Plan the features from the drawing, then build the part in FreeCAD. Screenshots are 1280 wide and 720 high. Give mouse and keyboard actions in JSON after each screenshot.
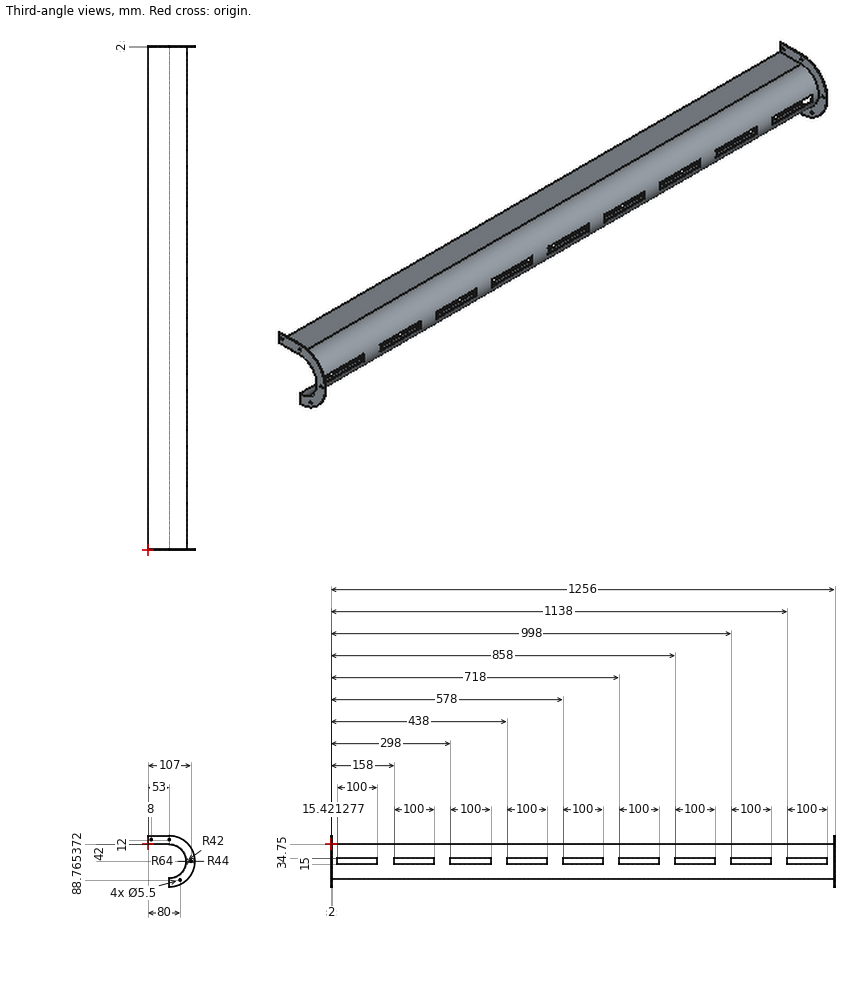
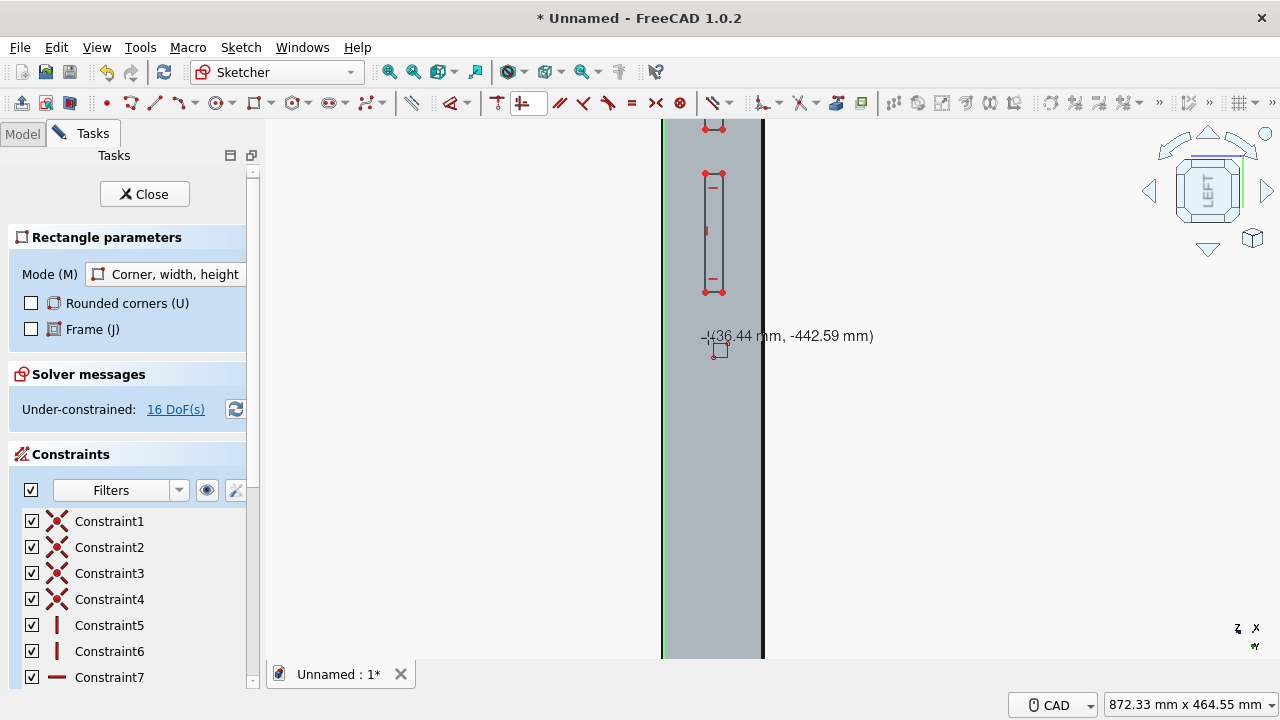
{"action": "left_click", "coordinate": [705, 335]}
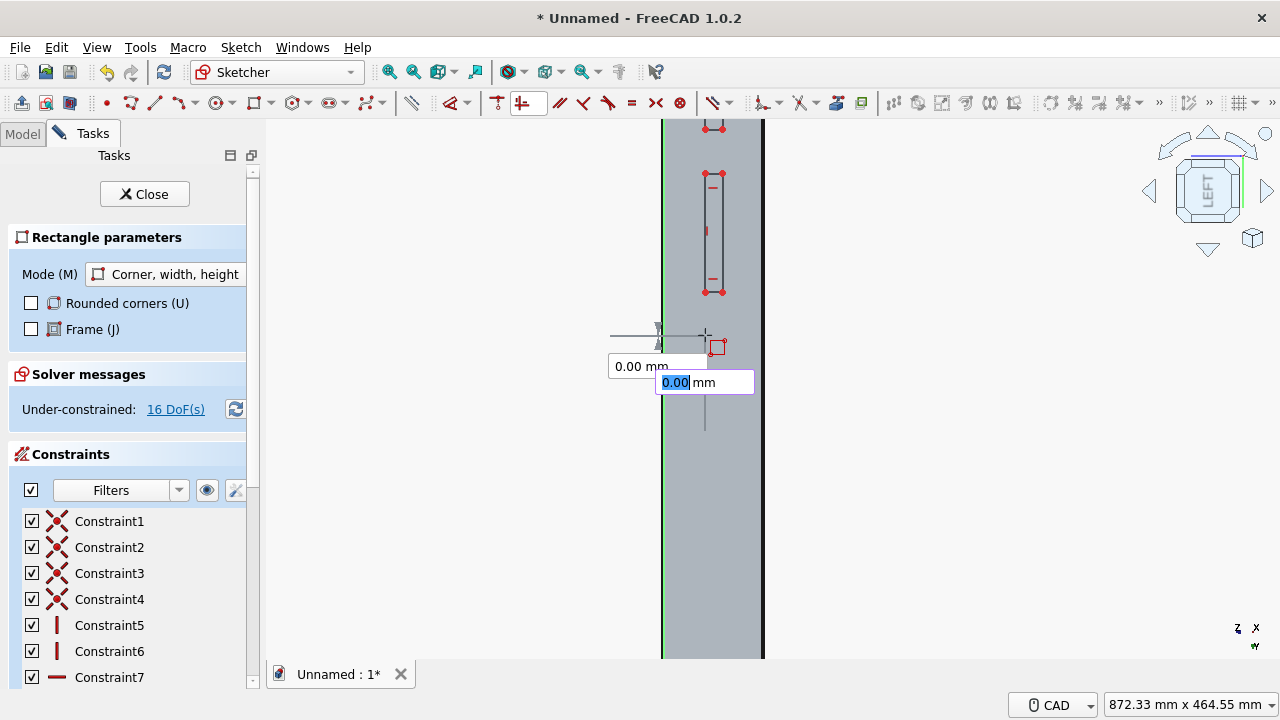
{"action": "scroll", "coordinate": [708, 338], "scroll_direction": "down", "scroll_amount": 7}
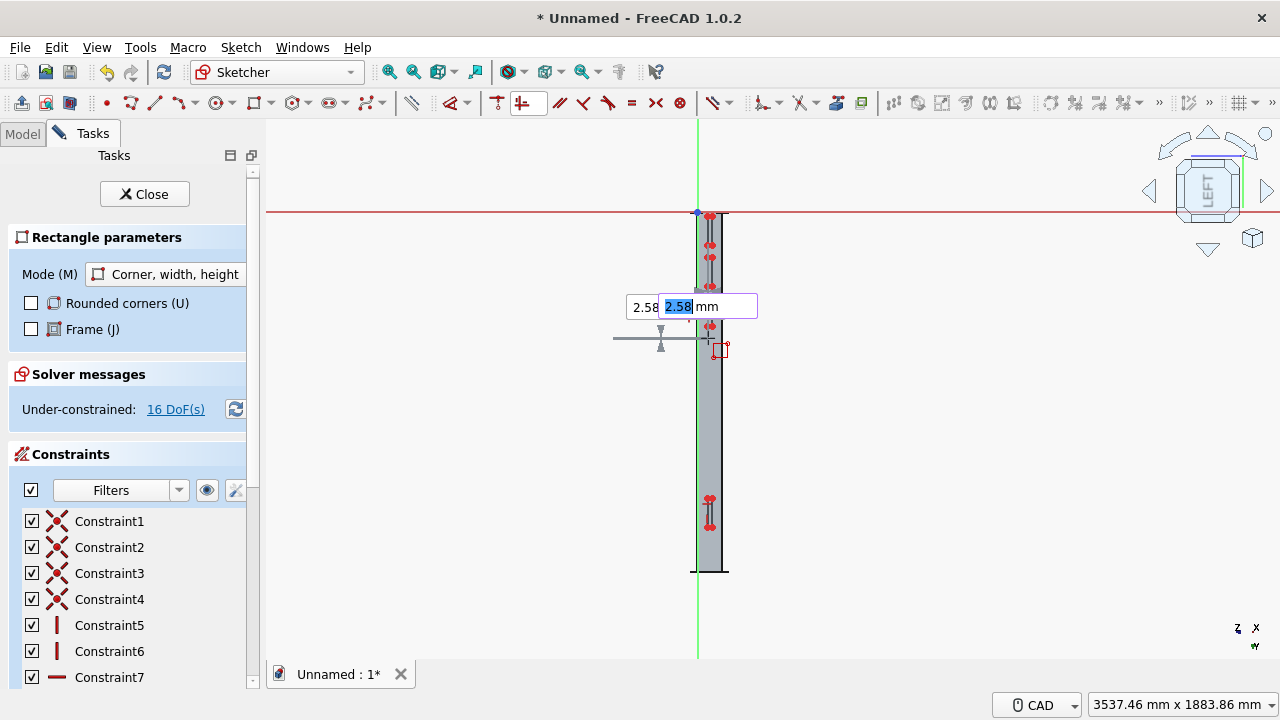
{"action": "left_click", "coordinate": [712, 366]}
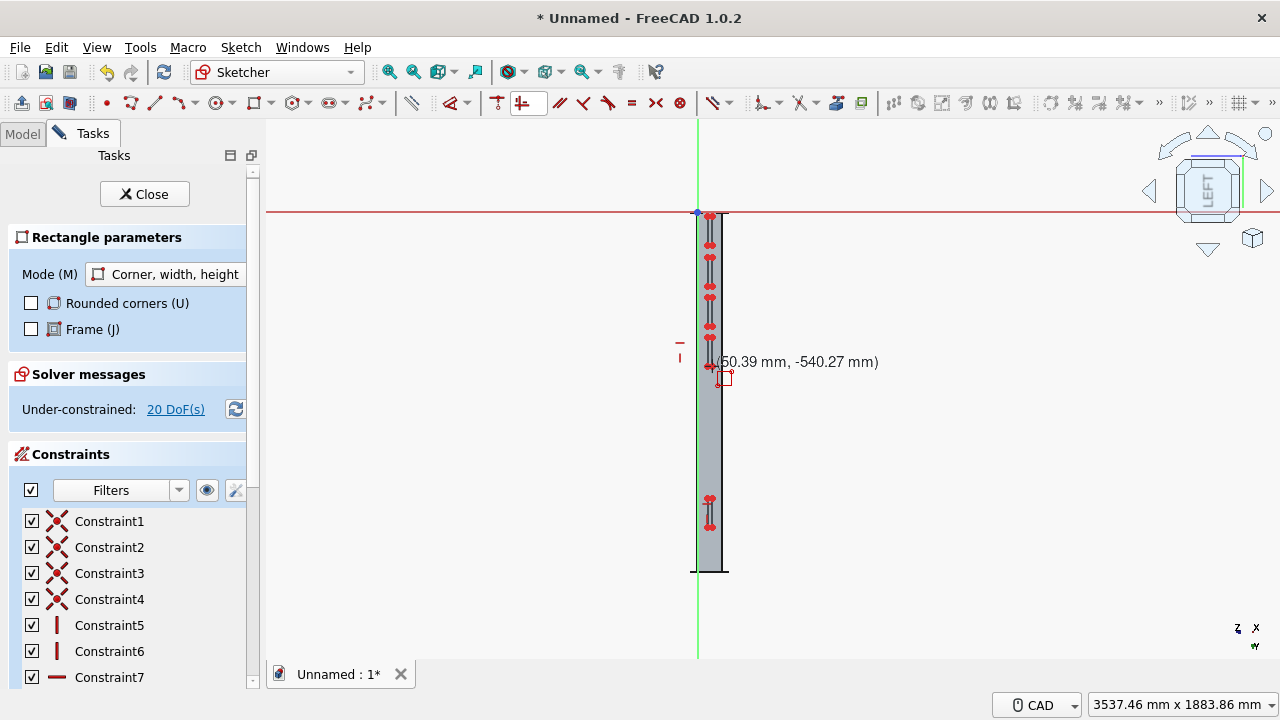
{"action": "scroll", "coordinate": [708, 378], "scroll_direction": "up", "scroll_amount": 7}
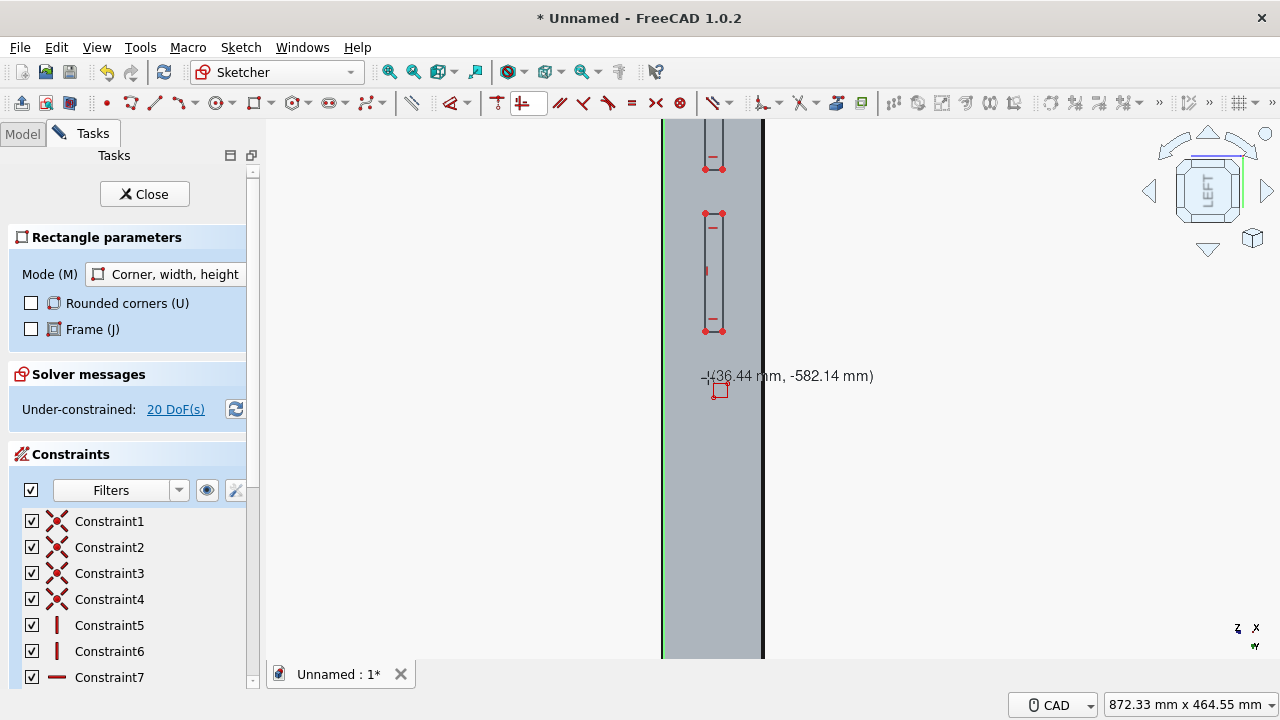
{"action": "left_click", "coordinate": [705, 376]}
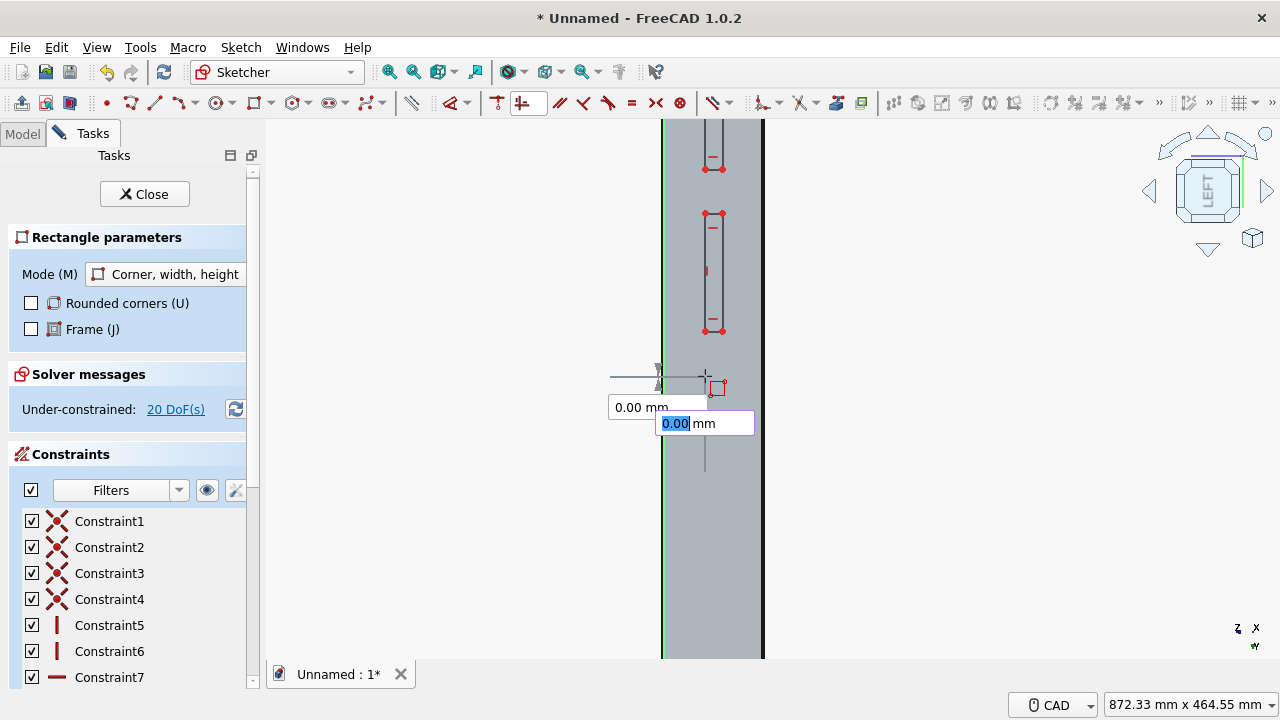
{"action": "scroll", "coordinate": [708, 378], "scroll_direction": "down", "scroll_amount": 7}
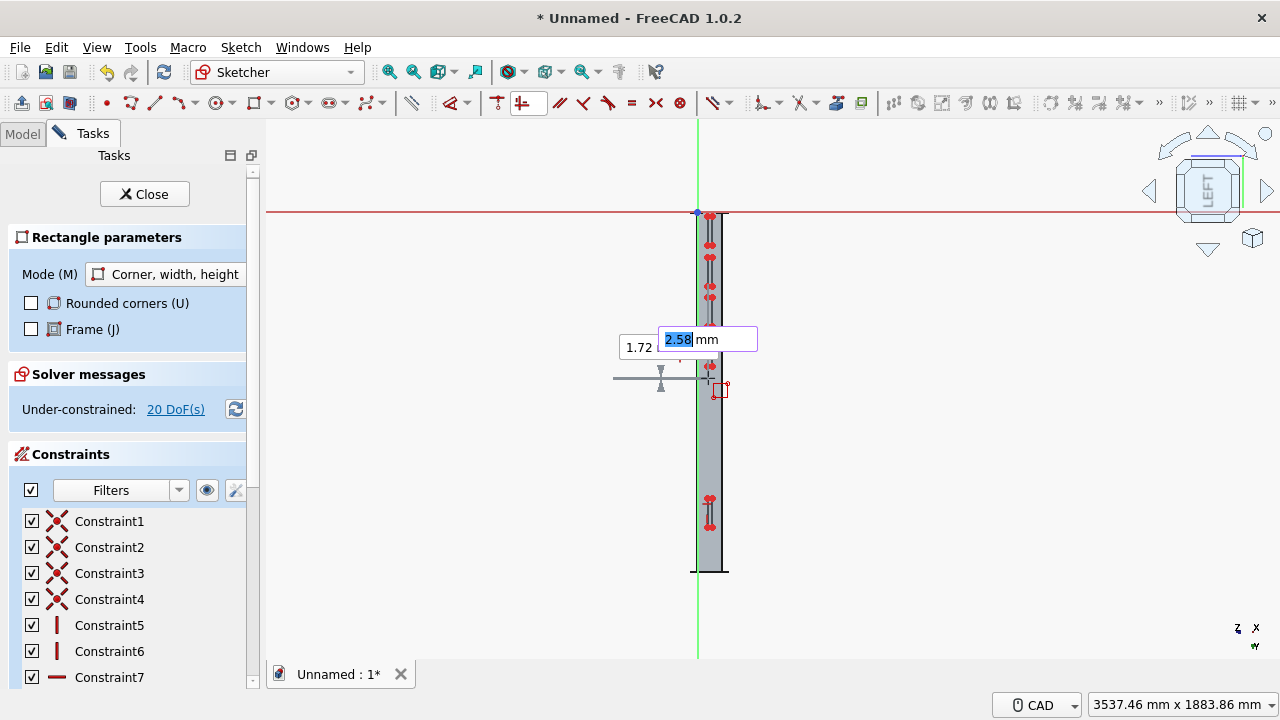
{"action": "left_click", "coordinate": [712, 406]}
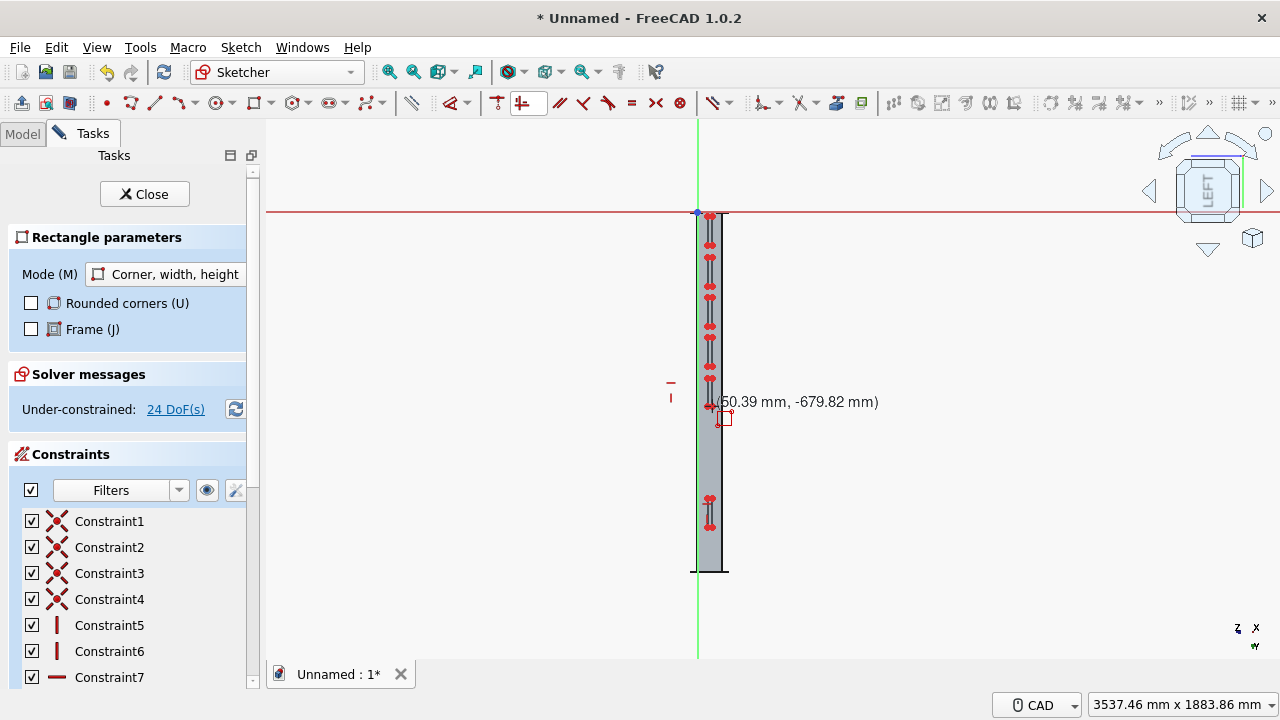
{"action": "scroll", "coordinate": [708, 418], "scroll_direction": "up", "scroll_amount": 7}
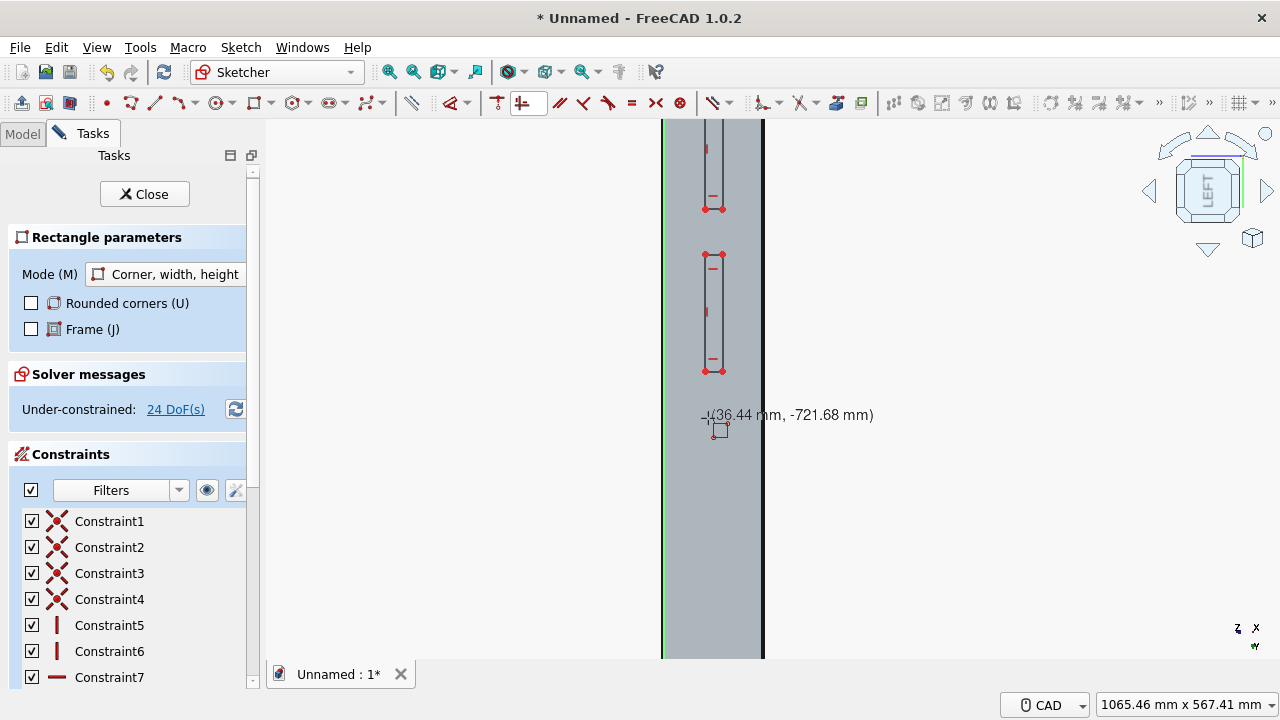
{"action": "left_click", "coordinate": [705, 416]}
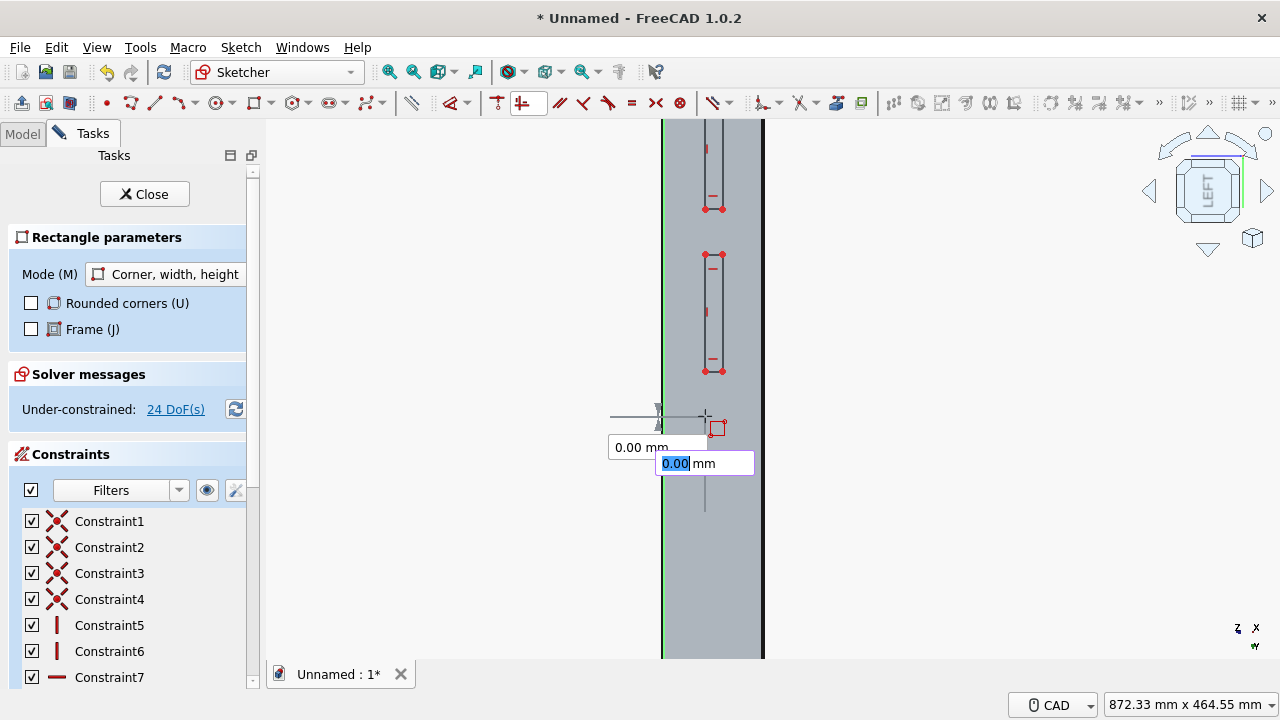
{"action": "scroll", "coordinate": [708, 418], "scroll_direction": "down", "scroll_amount": 7}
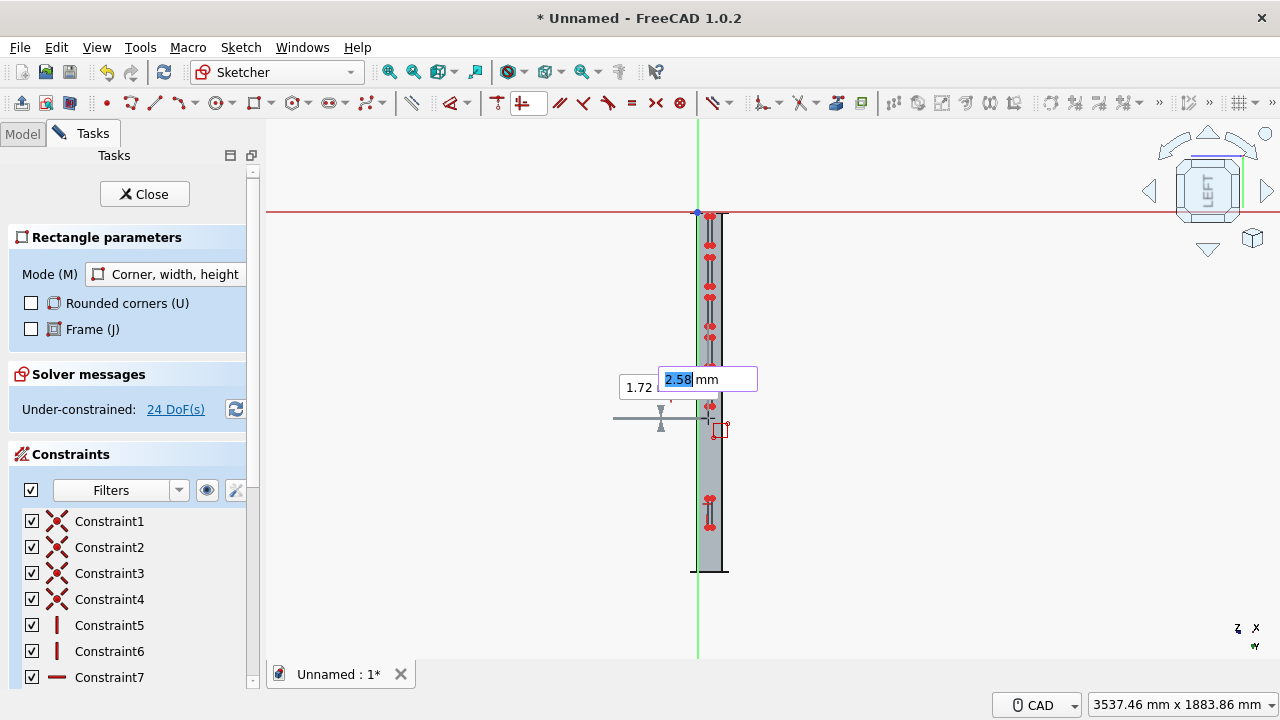
{"action": "left_click", "coordinate": [712, 447]}